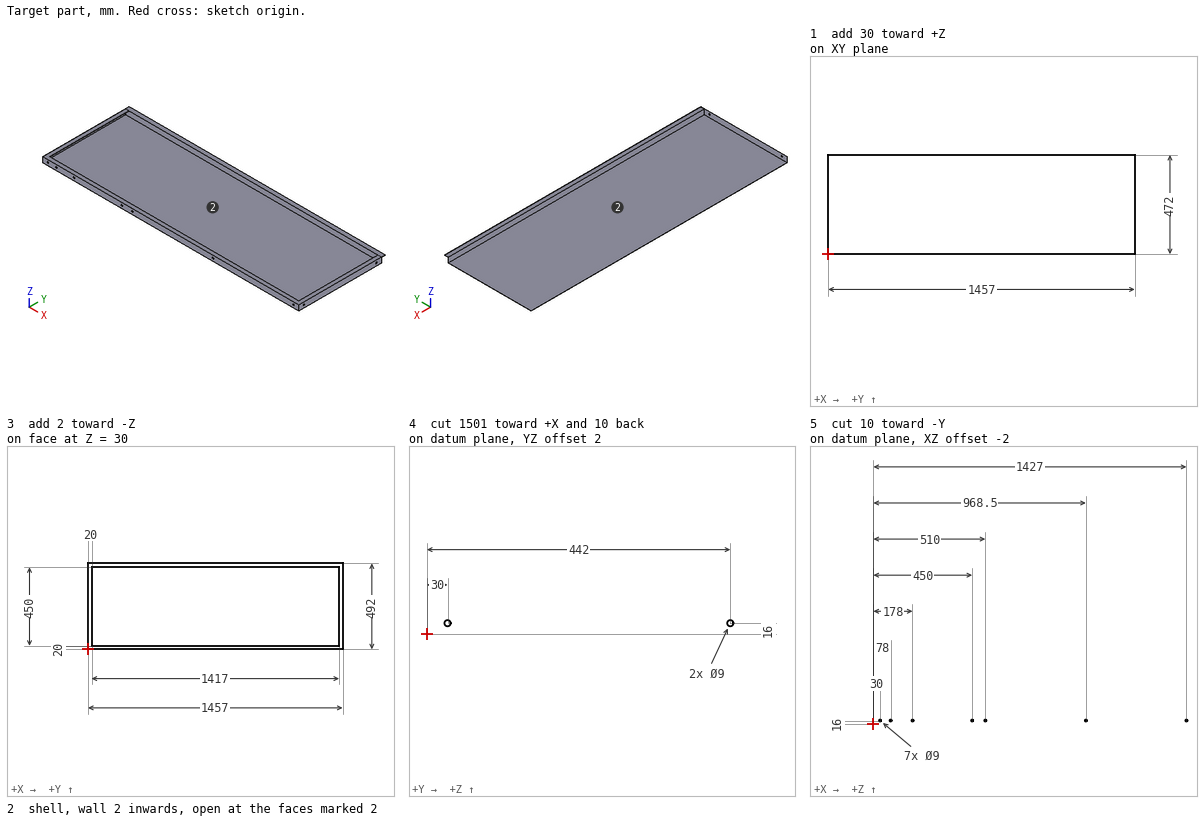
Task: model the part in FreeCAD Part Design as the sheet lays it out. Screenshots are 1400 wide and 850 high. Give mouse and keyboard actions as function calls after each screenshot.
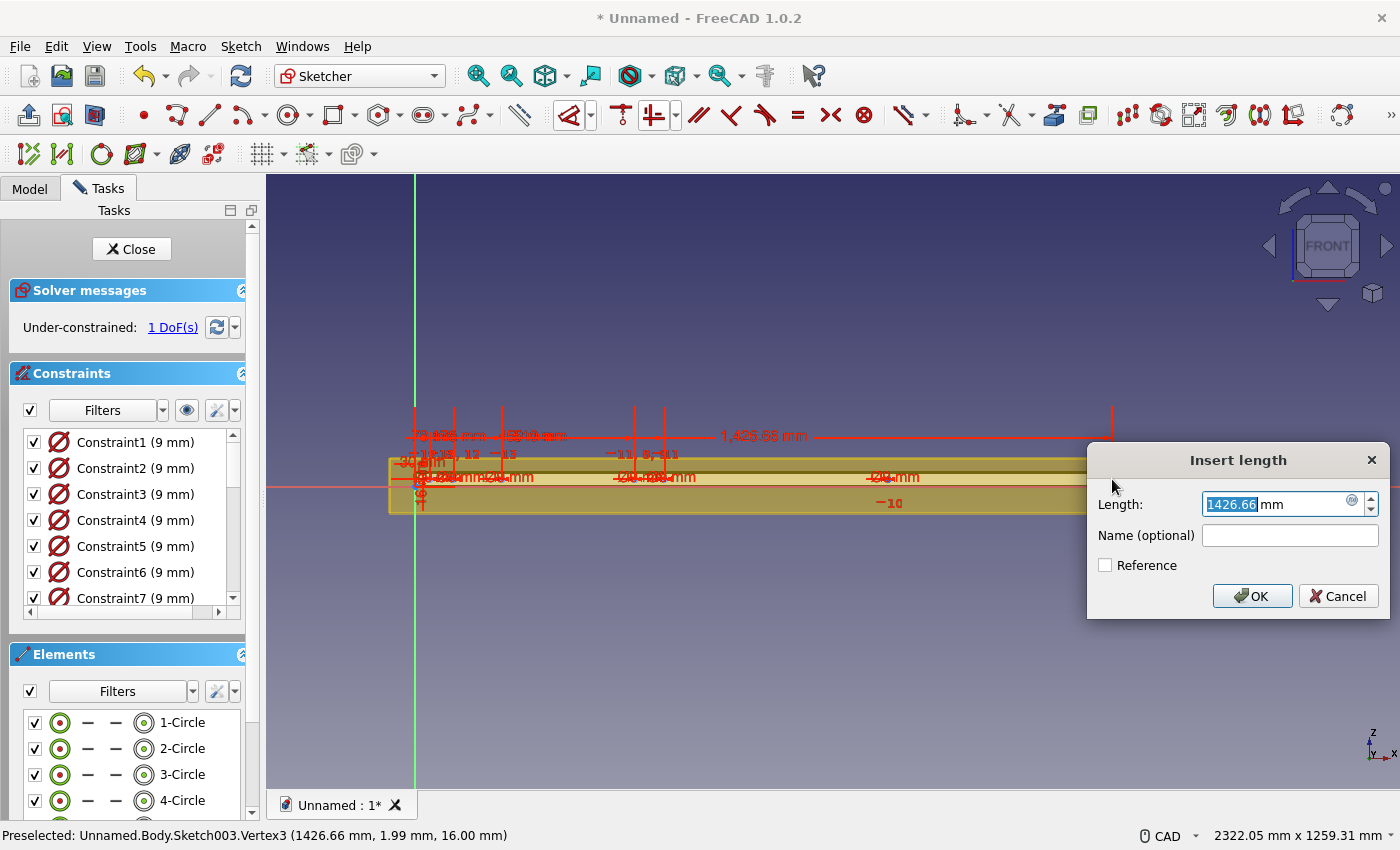
text(1427)
key(Return)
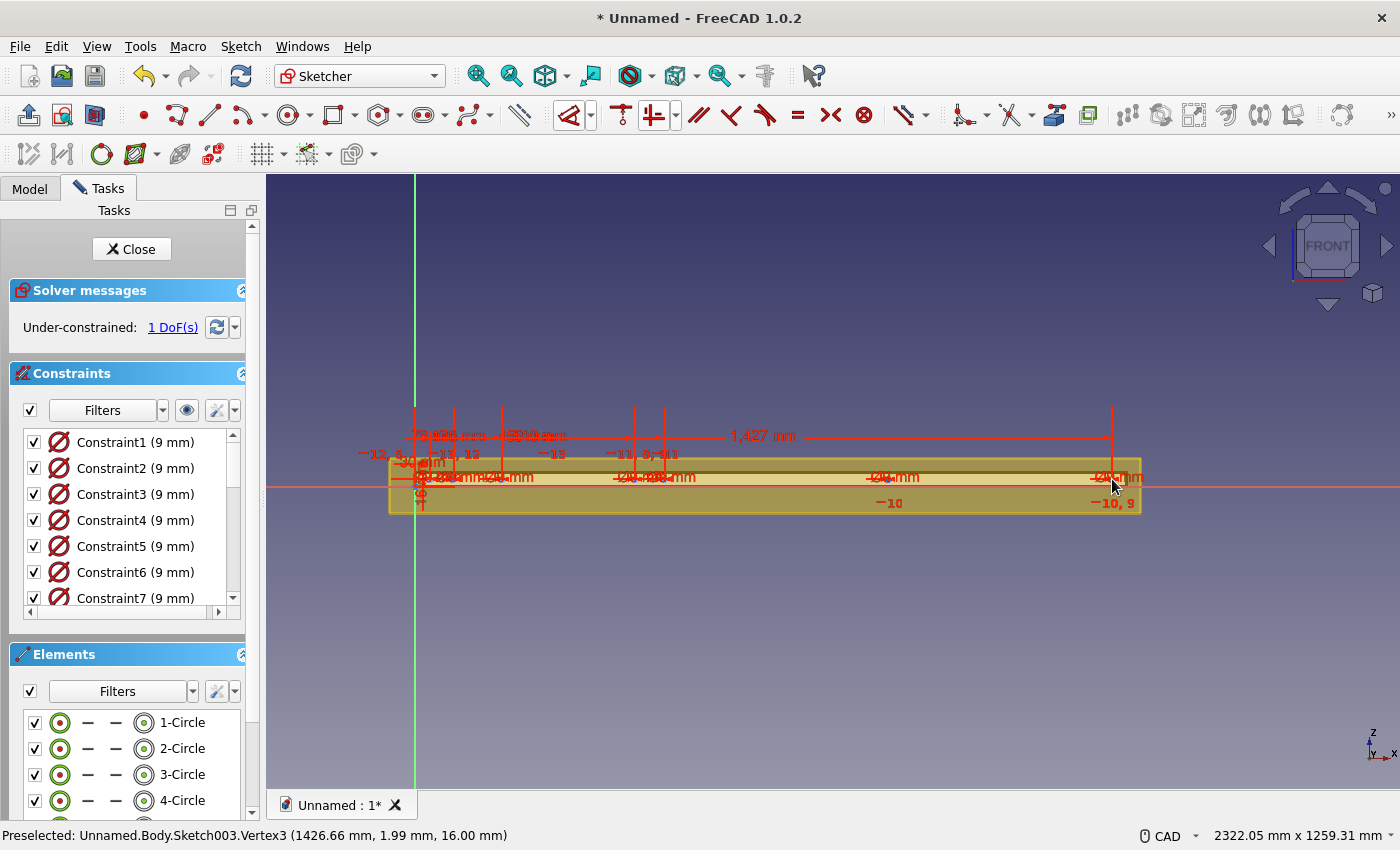
click(888, 479)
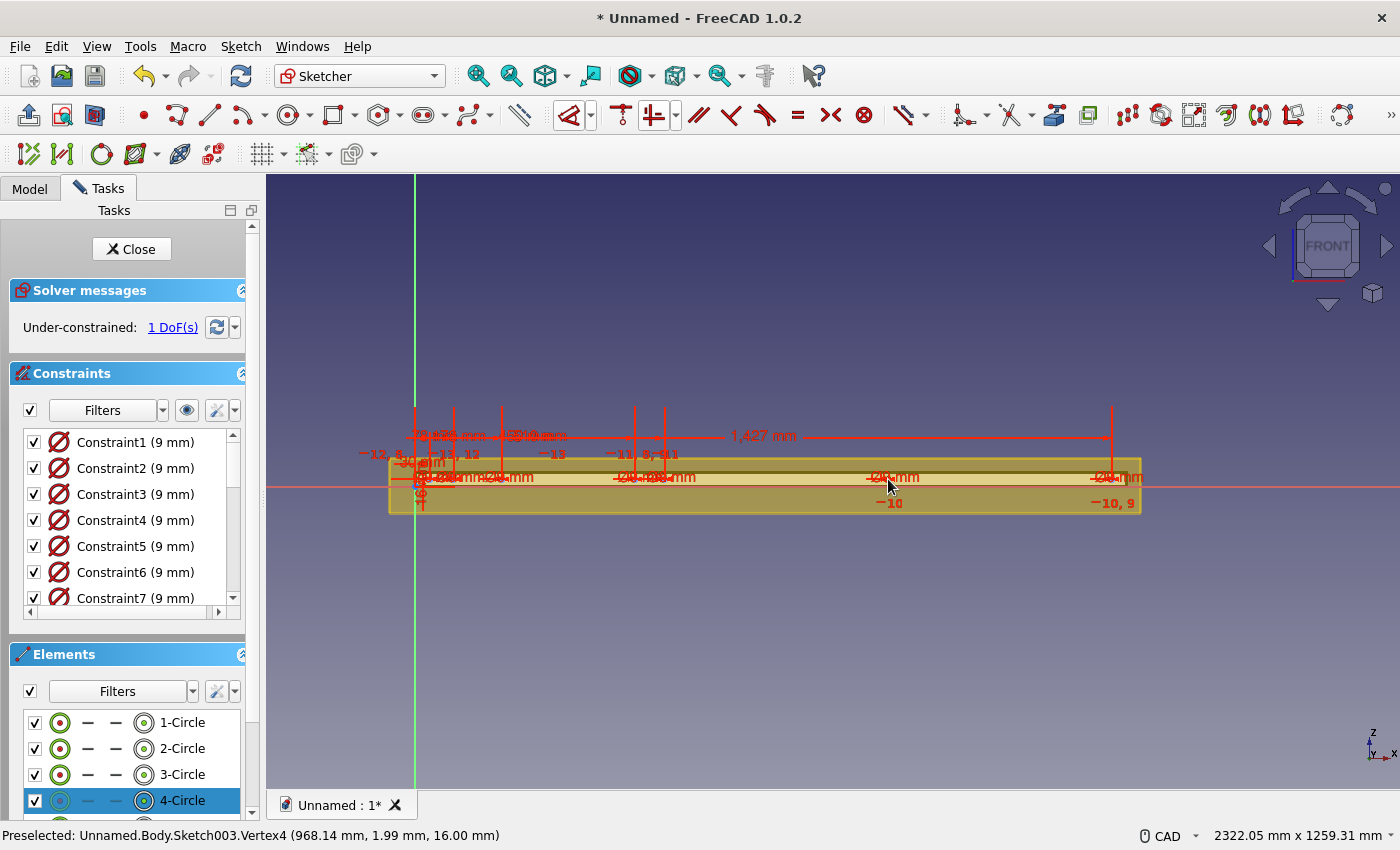
key(l)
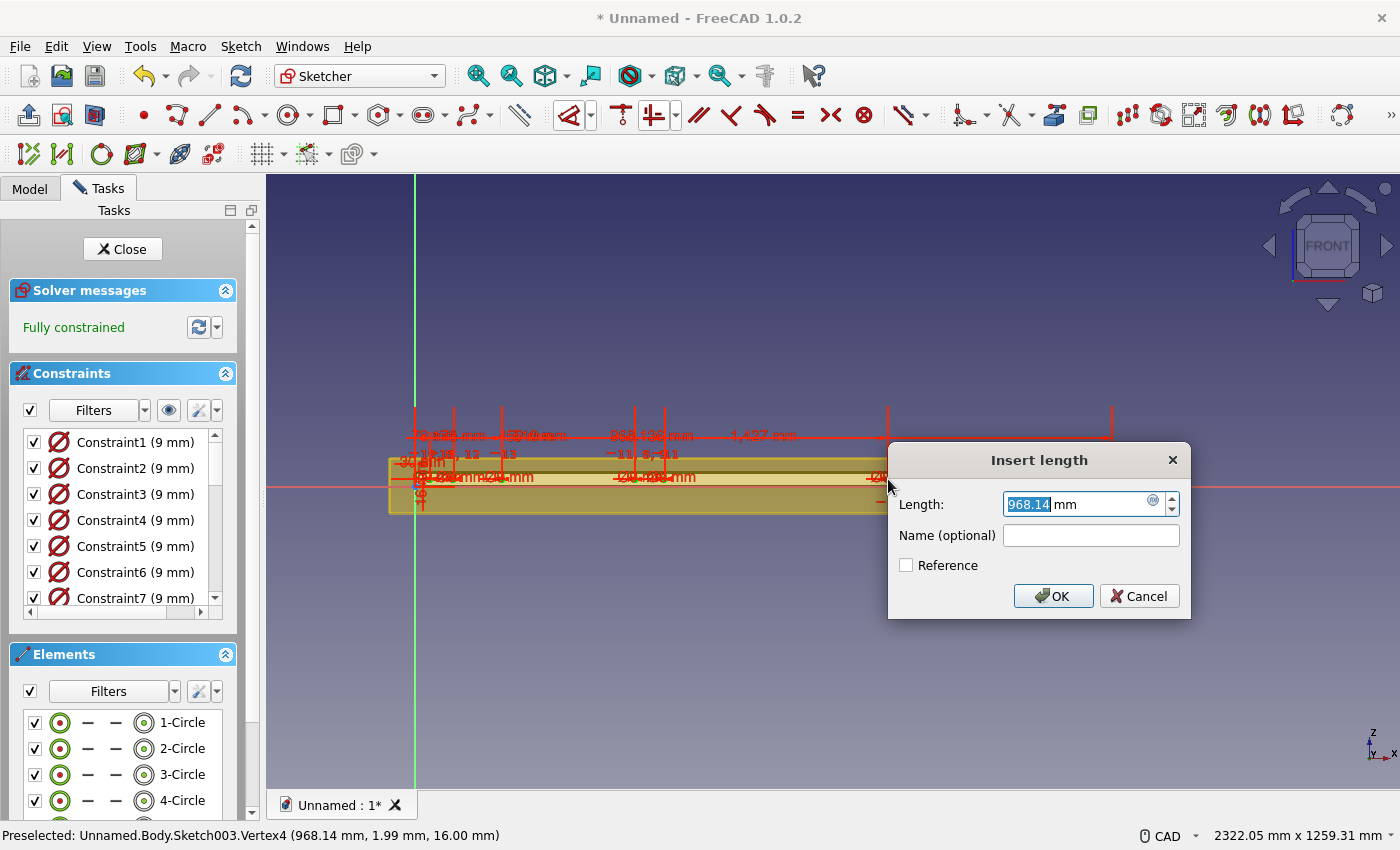
text(968.5)
key(Return)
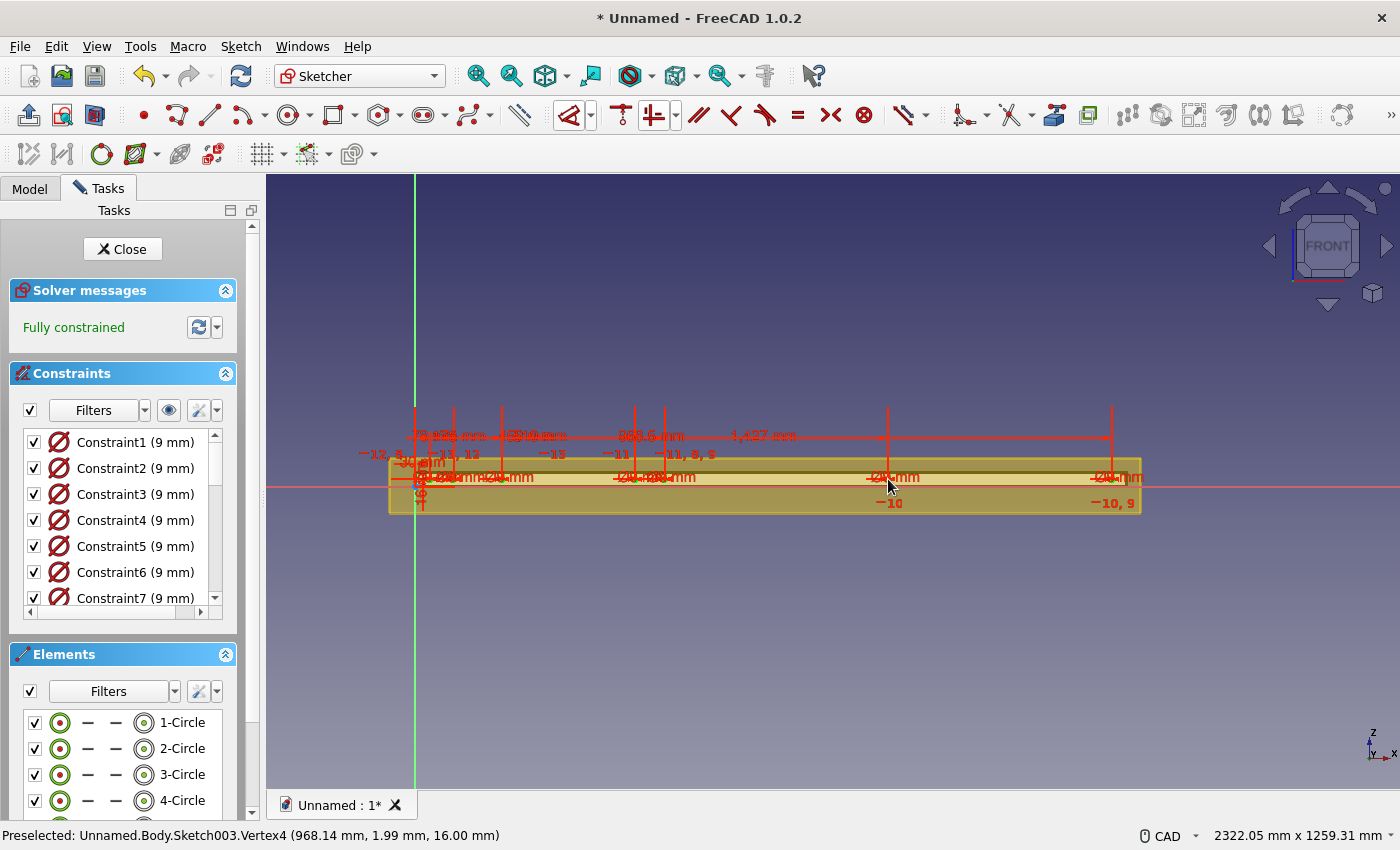
click(123, 249)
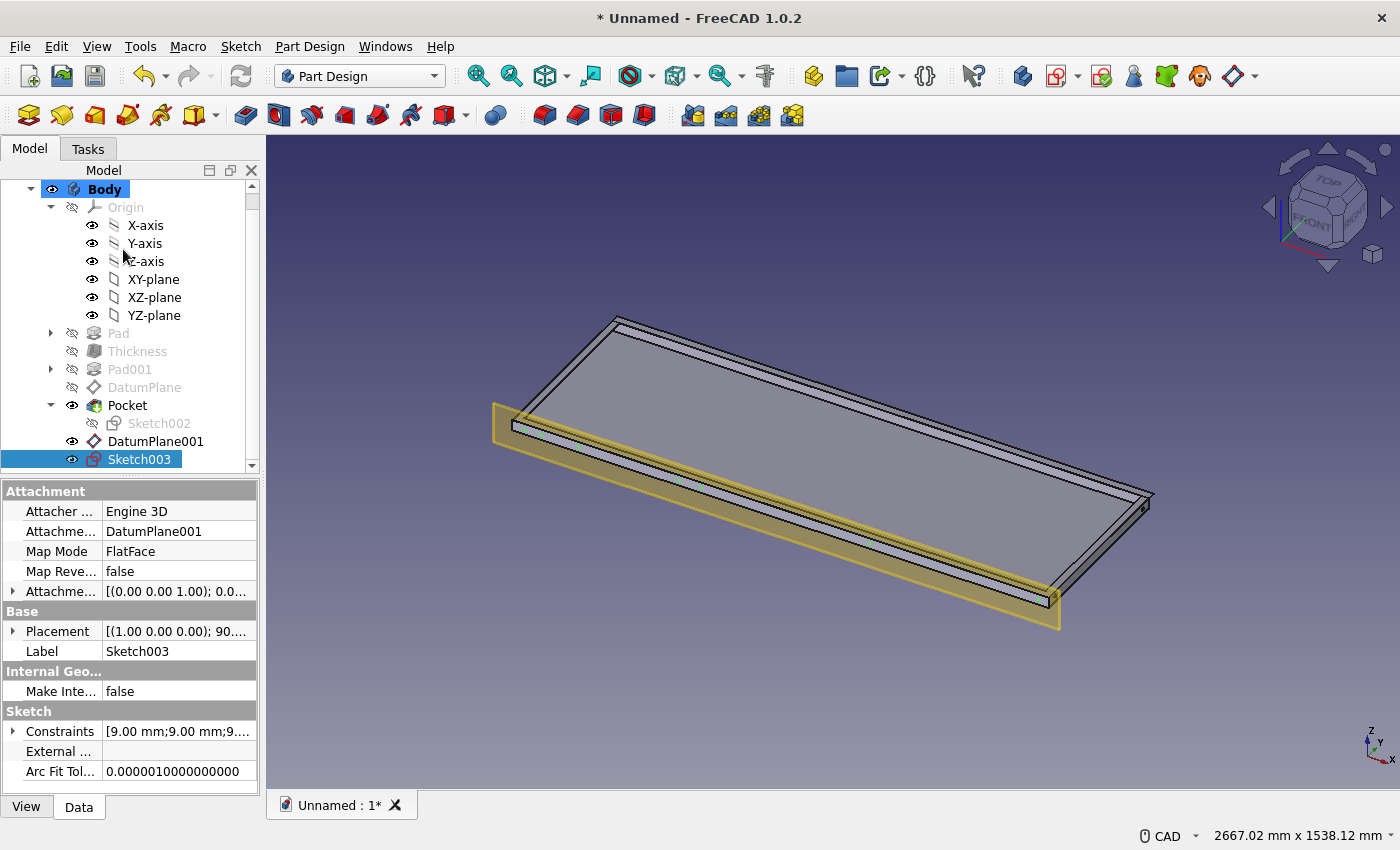
click(246, 116)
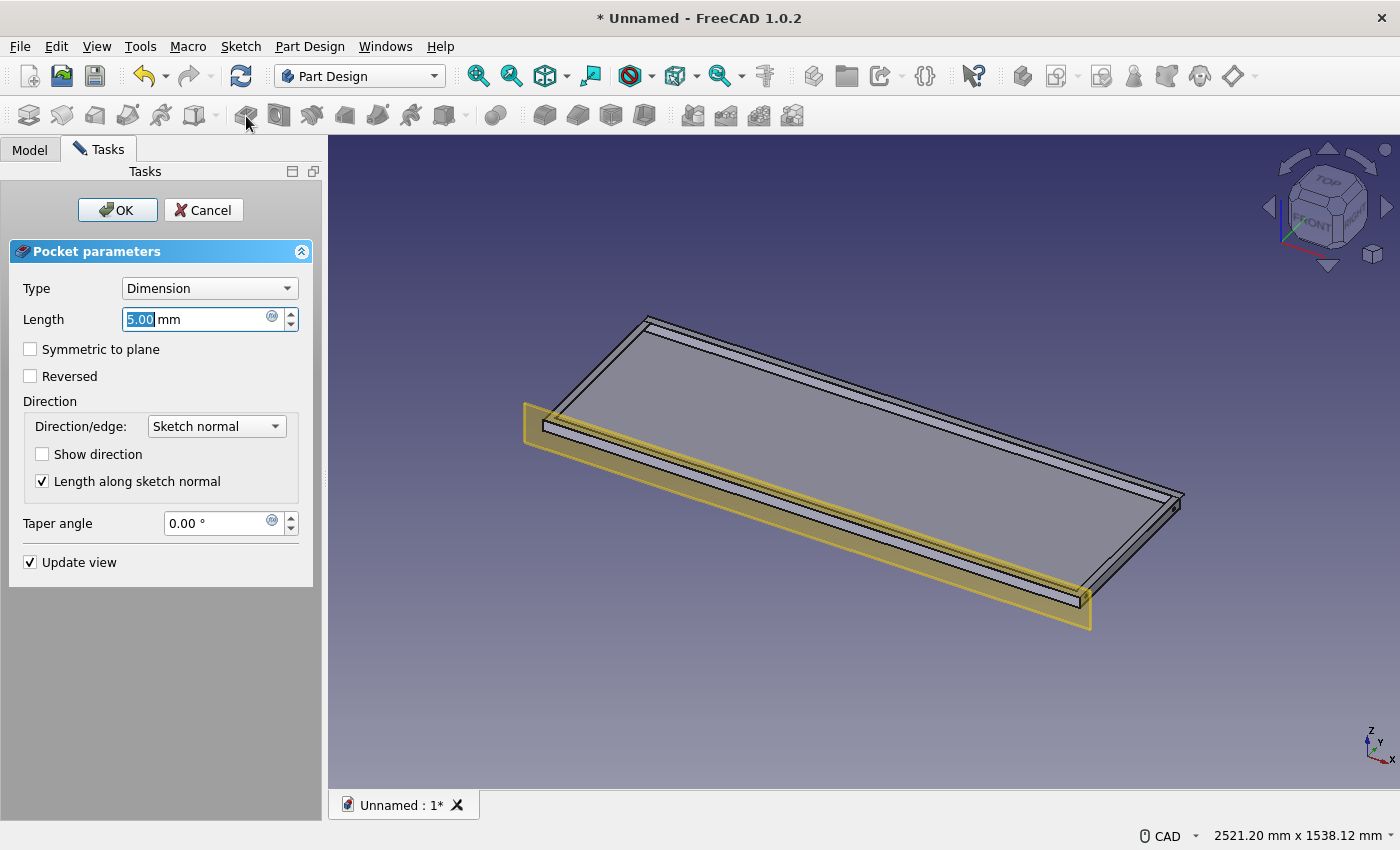
text(10)
key(Tab)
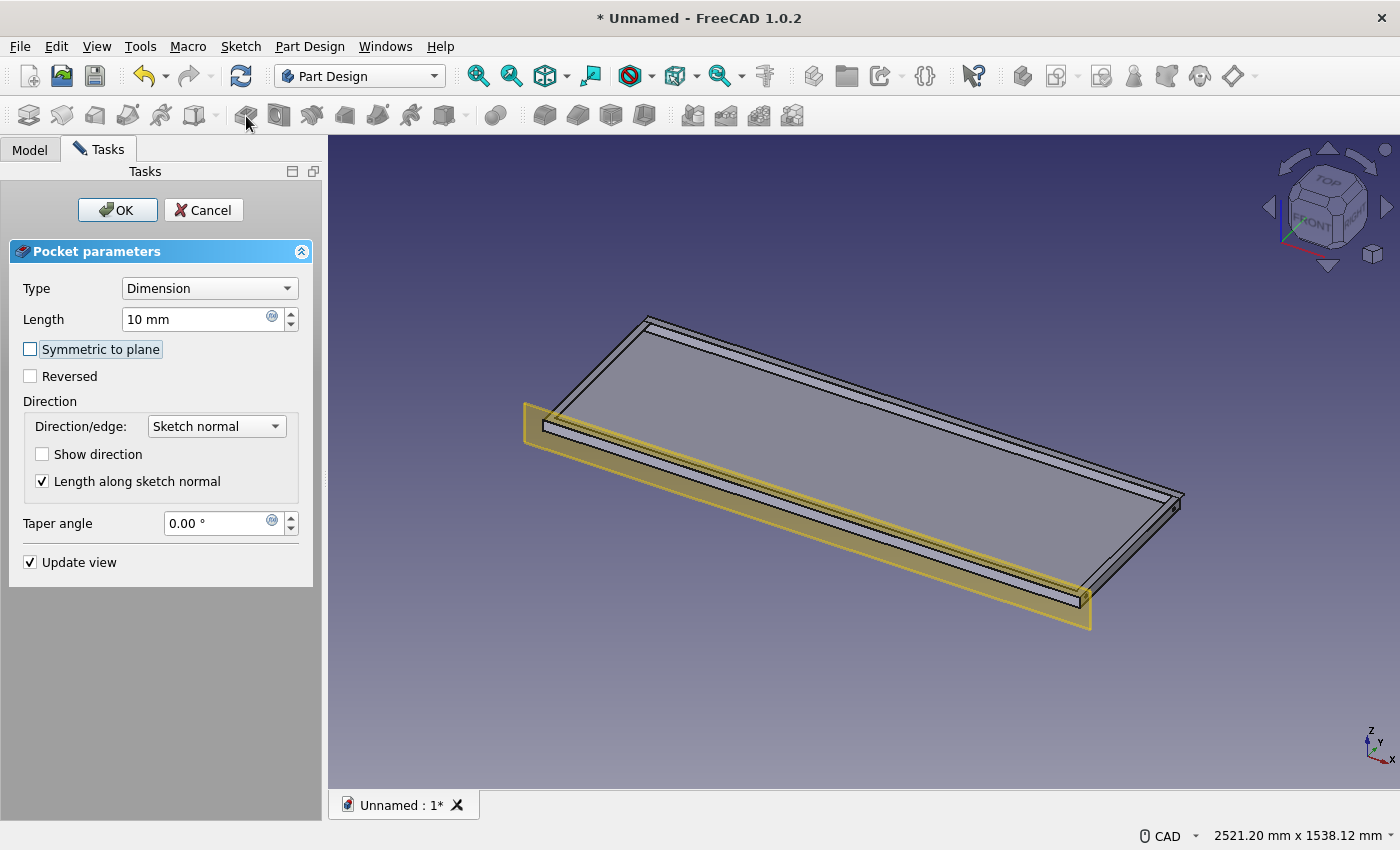
click(31, 376)